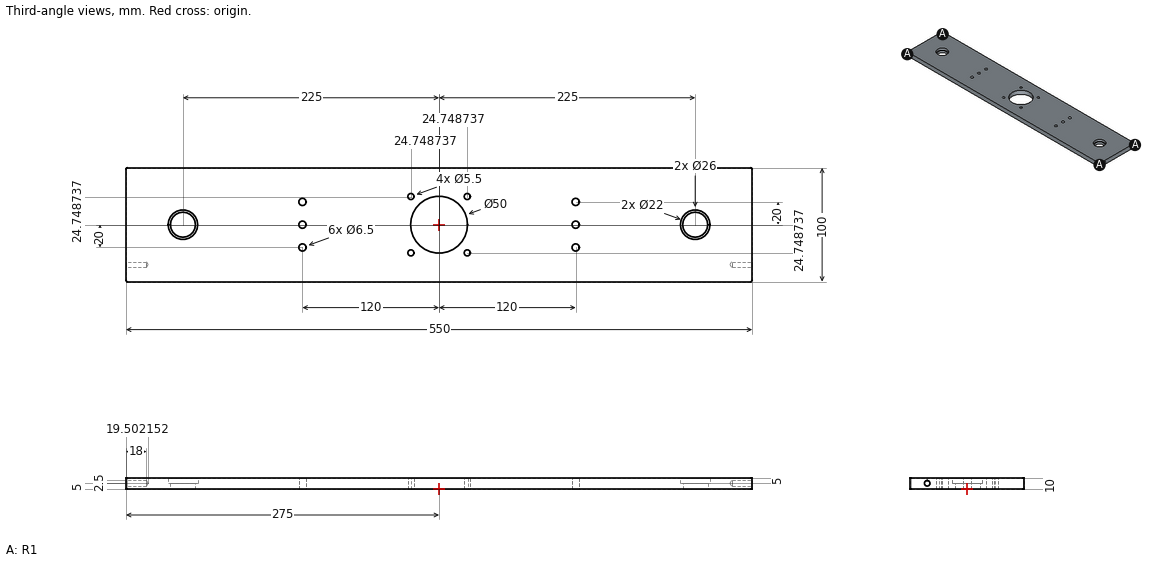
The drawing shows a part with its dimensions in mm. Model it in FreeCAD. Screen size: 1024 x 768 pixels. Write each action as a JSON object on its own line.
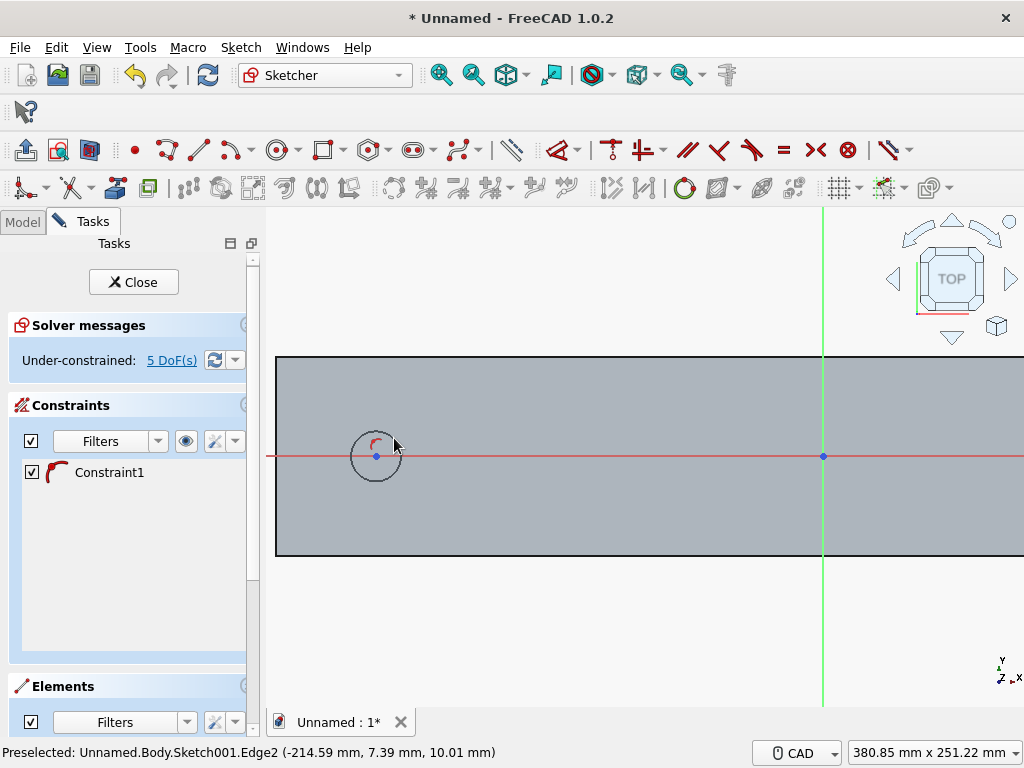
{"action": "scroll", "coordinate": [375, 458], "scroll_direction": "down", "scroll_amount": 4}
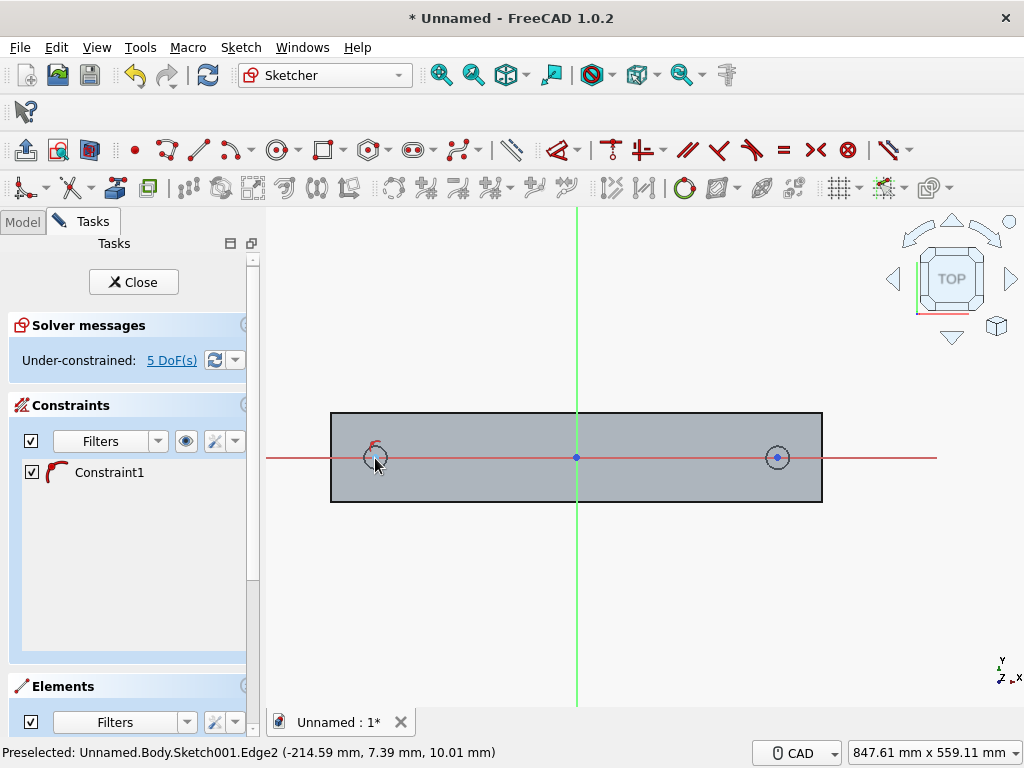
{"action": "scroll", "coordinate": [786, 450], "scroll_direction": "up", "scroll_amount": 3}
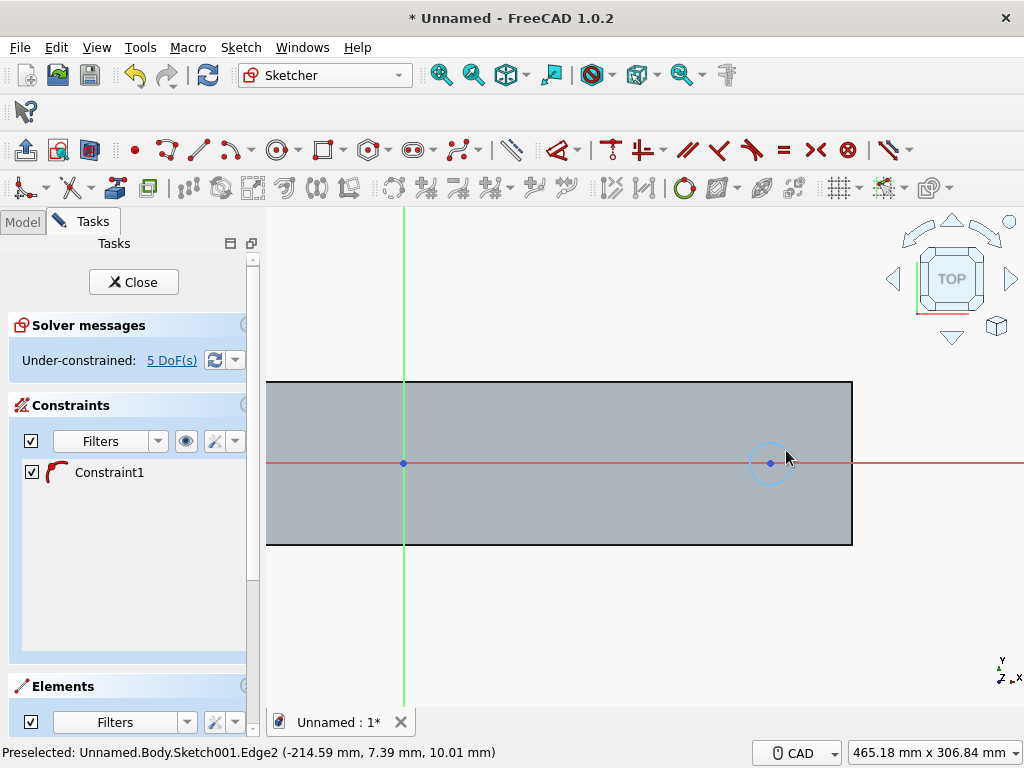
{"action": "left_click", "coordinate": [785, 449]}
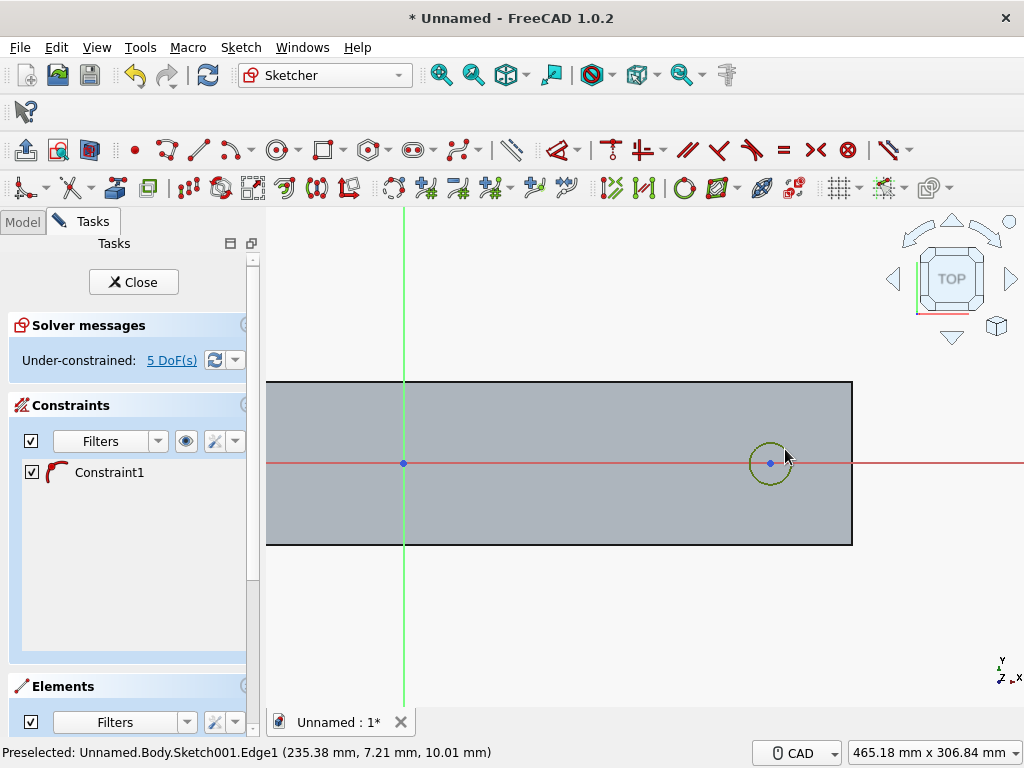
{"action": "scroll", "coordinate": [787, 449], "scroll_direction": "down", "scroll_amount": 3}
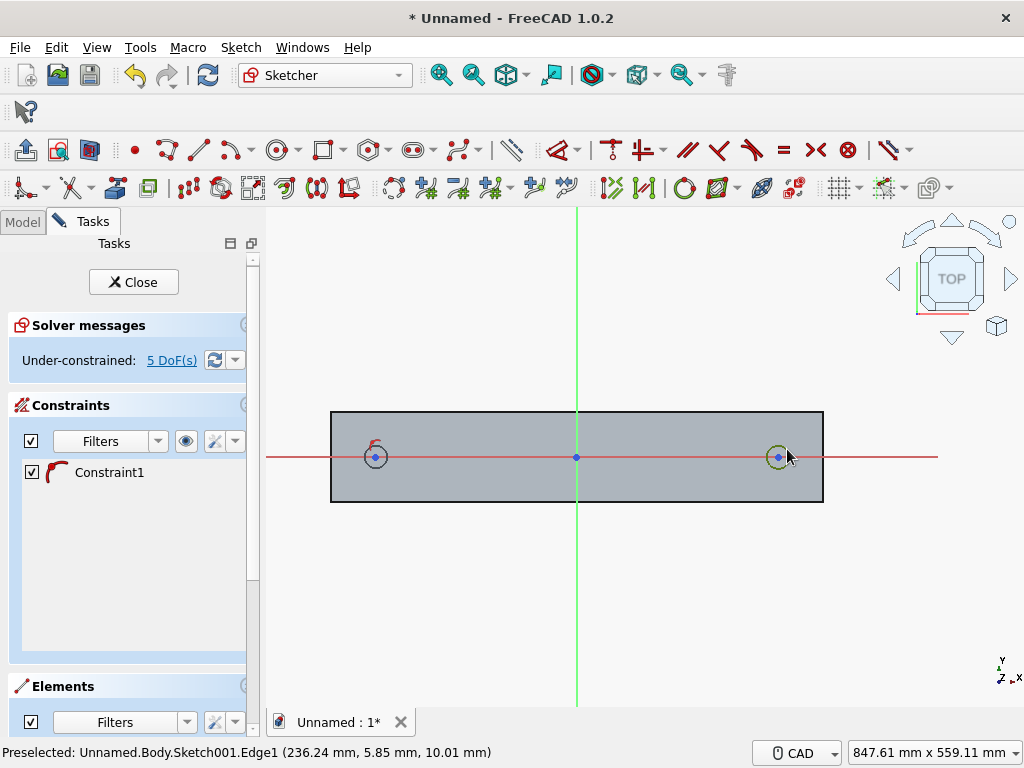
{"action": "scroll", "coordinate": [384, 449], "scroll_direction": "up", "scroll_amount": 3}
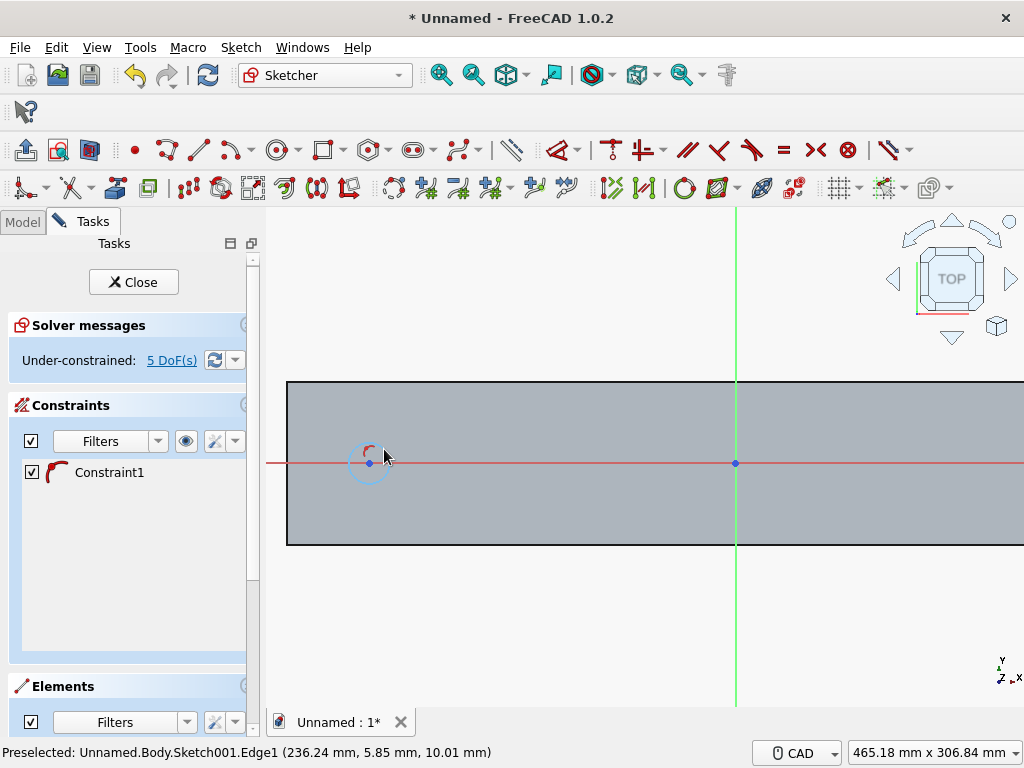
{"action": "left_click", "coordinate": [384, 449]}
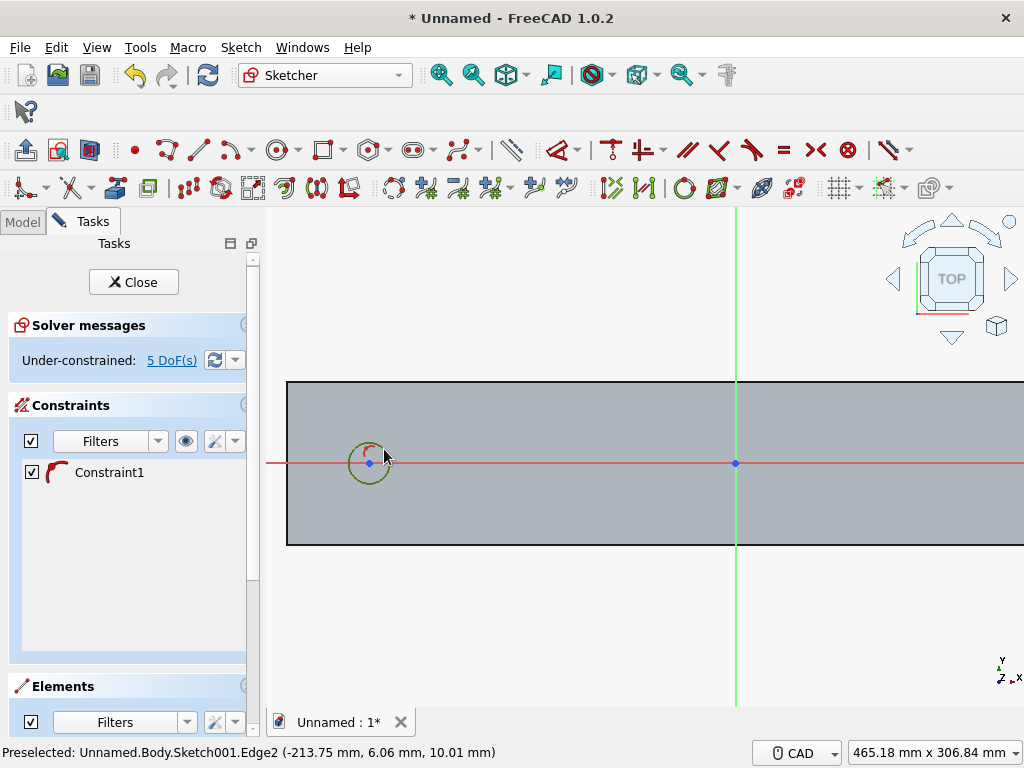
{"action": "key", "text": "e"}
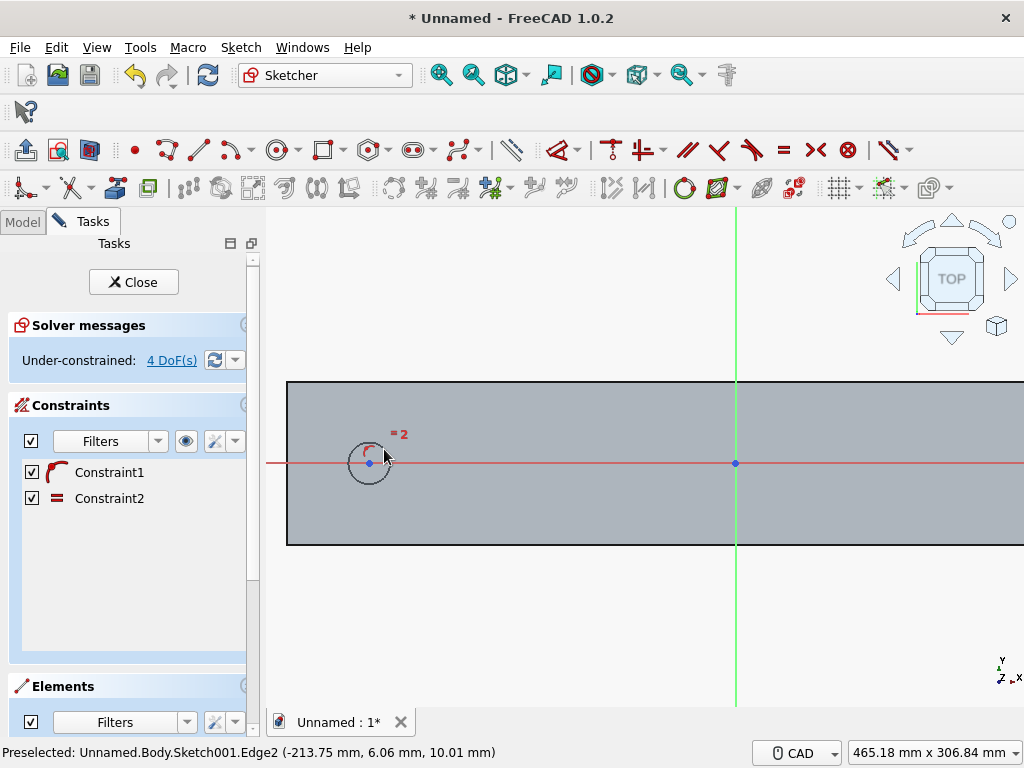
{"action": "scroll", "coordinate": [383, 449], "scroll_direction": "down", "scroll_amount": 3}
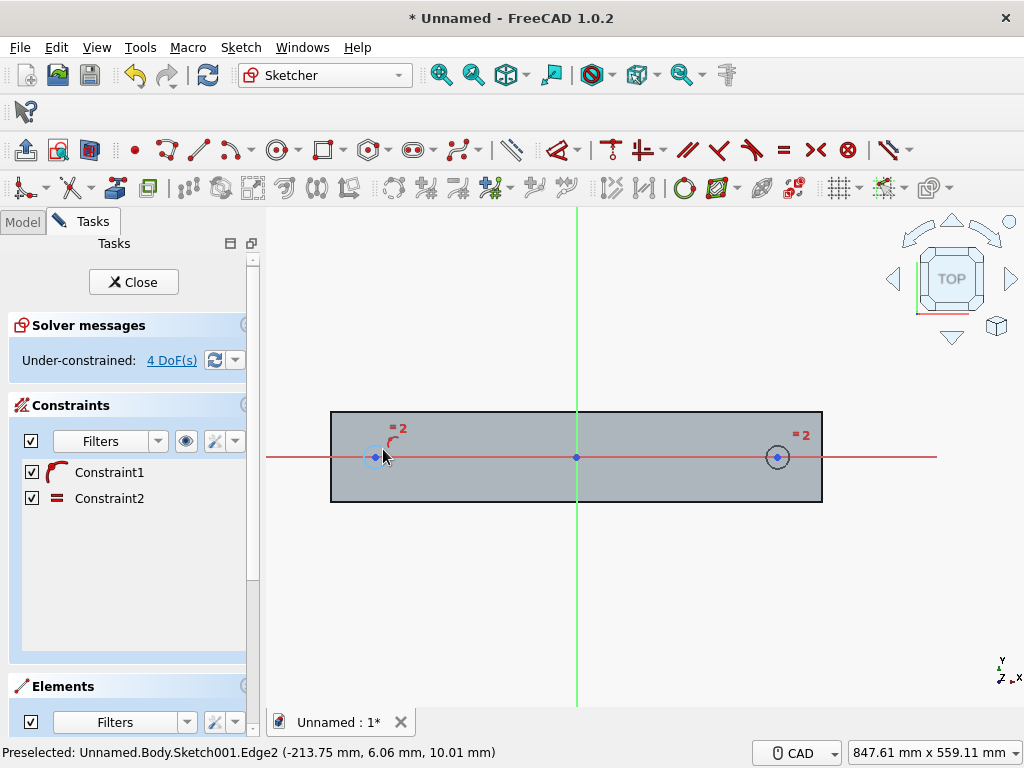
{"action": "left_click", "coordinate": [778, 457]}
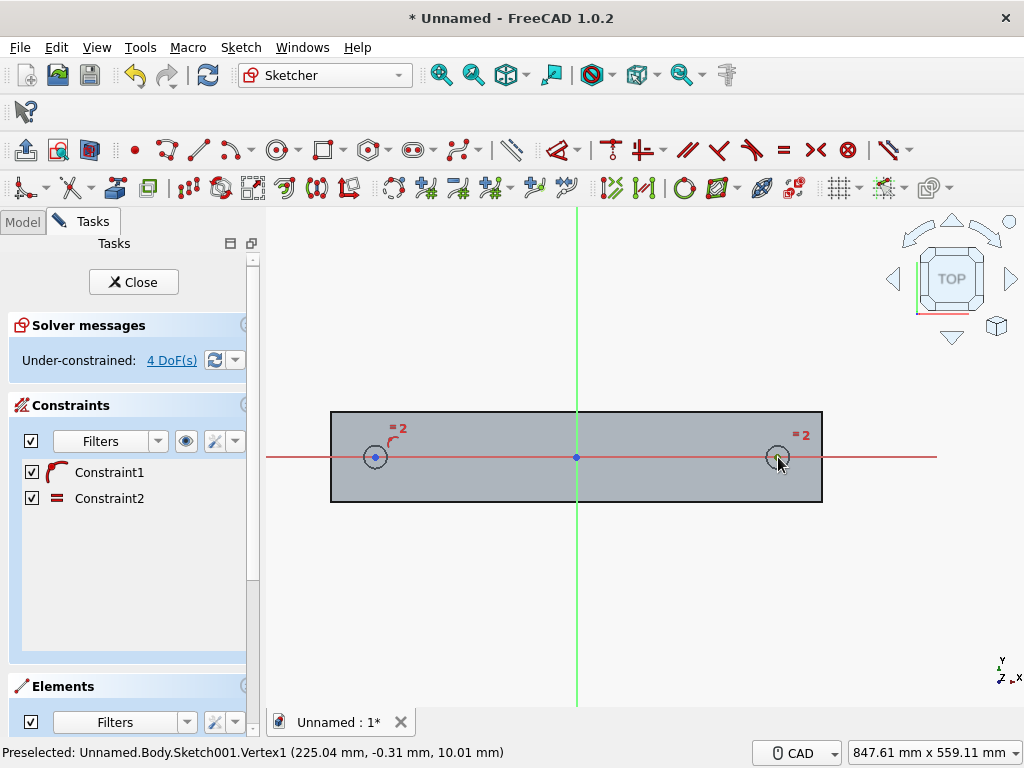
{"action": "left_click", "coordinate": [455, 457]}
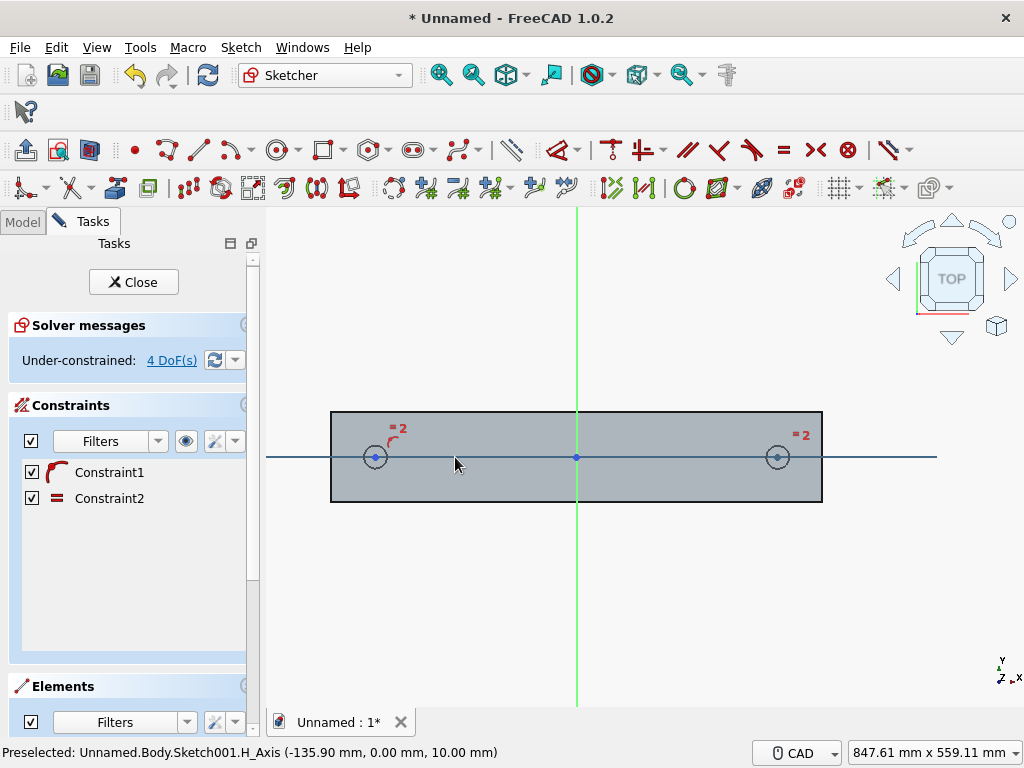
{"action": "left_click", "coordinate": [612, 150]}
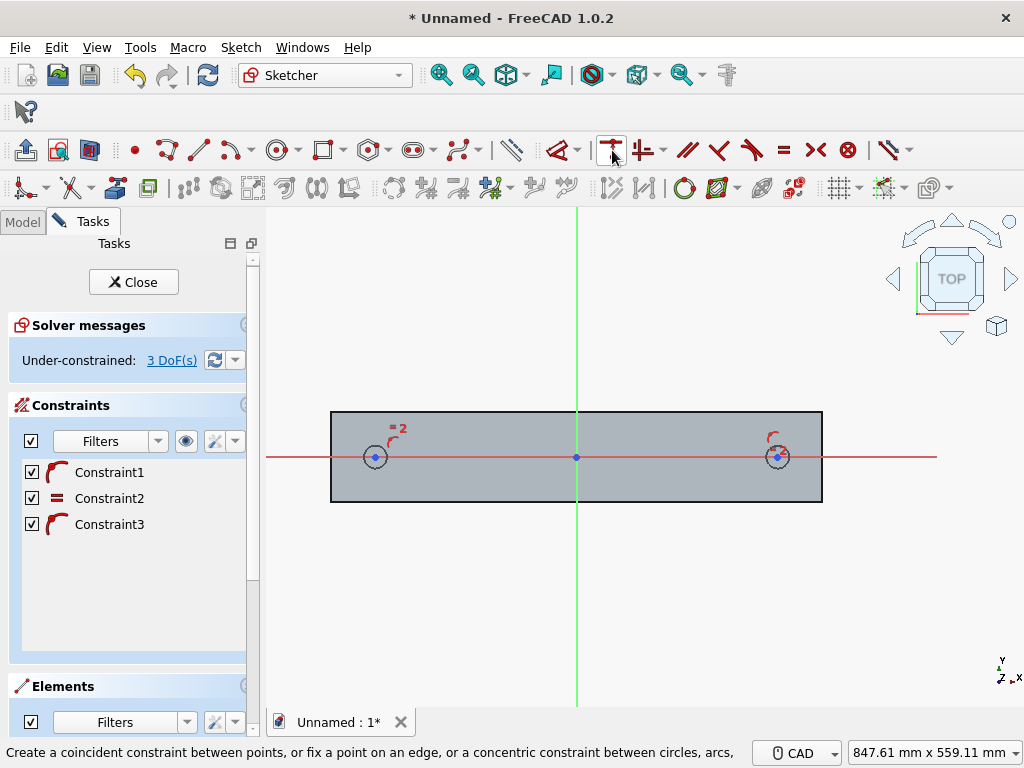
{"action": "key", "text": "d"}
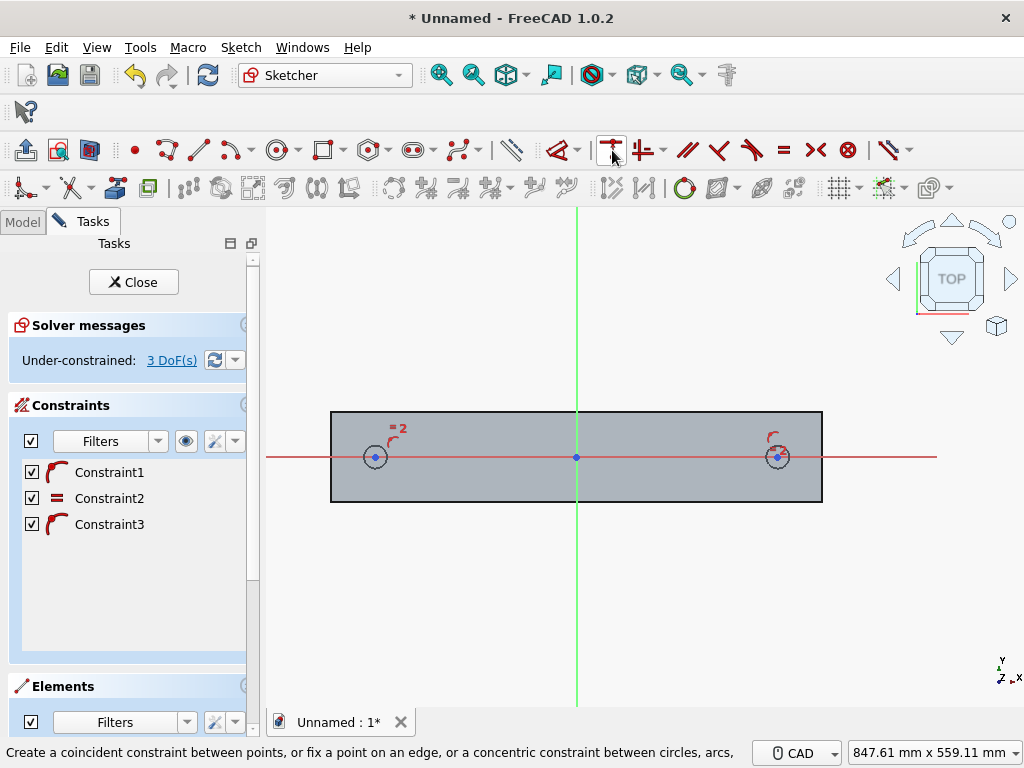
{"action": "scroll", "coordinate": [778, 446], "scroll_direction": "up", "scroll_amount": 3}